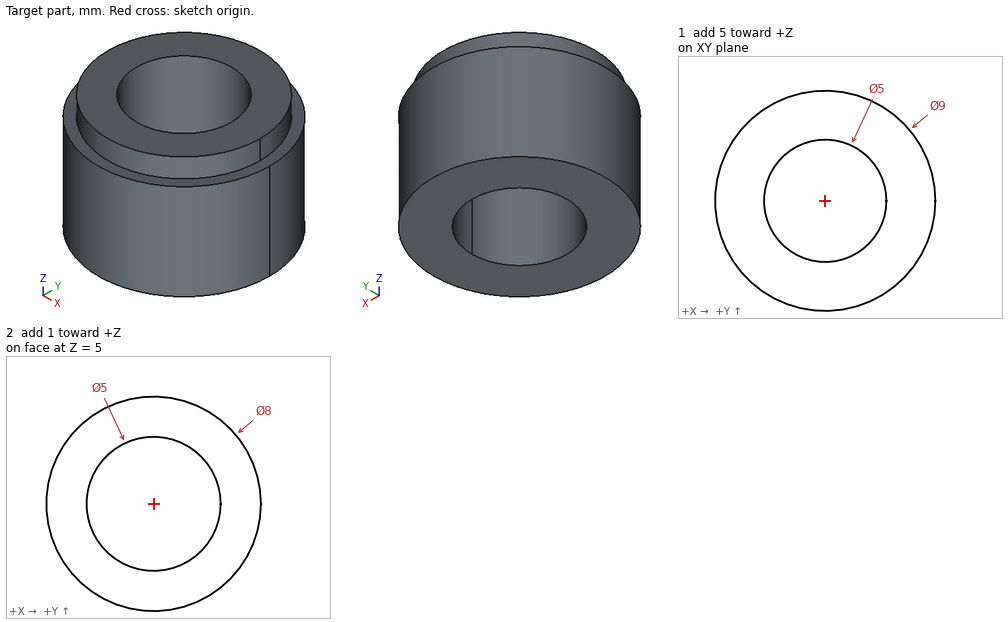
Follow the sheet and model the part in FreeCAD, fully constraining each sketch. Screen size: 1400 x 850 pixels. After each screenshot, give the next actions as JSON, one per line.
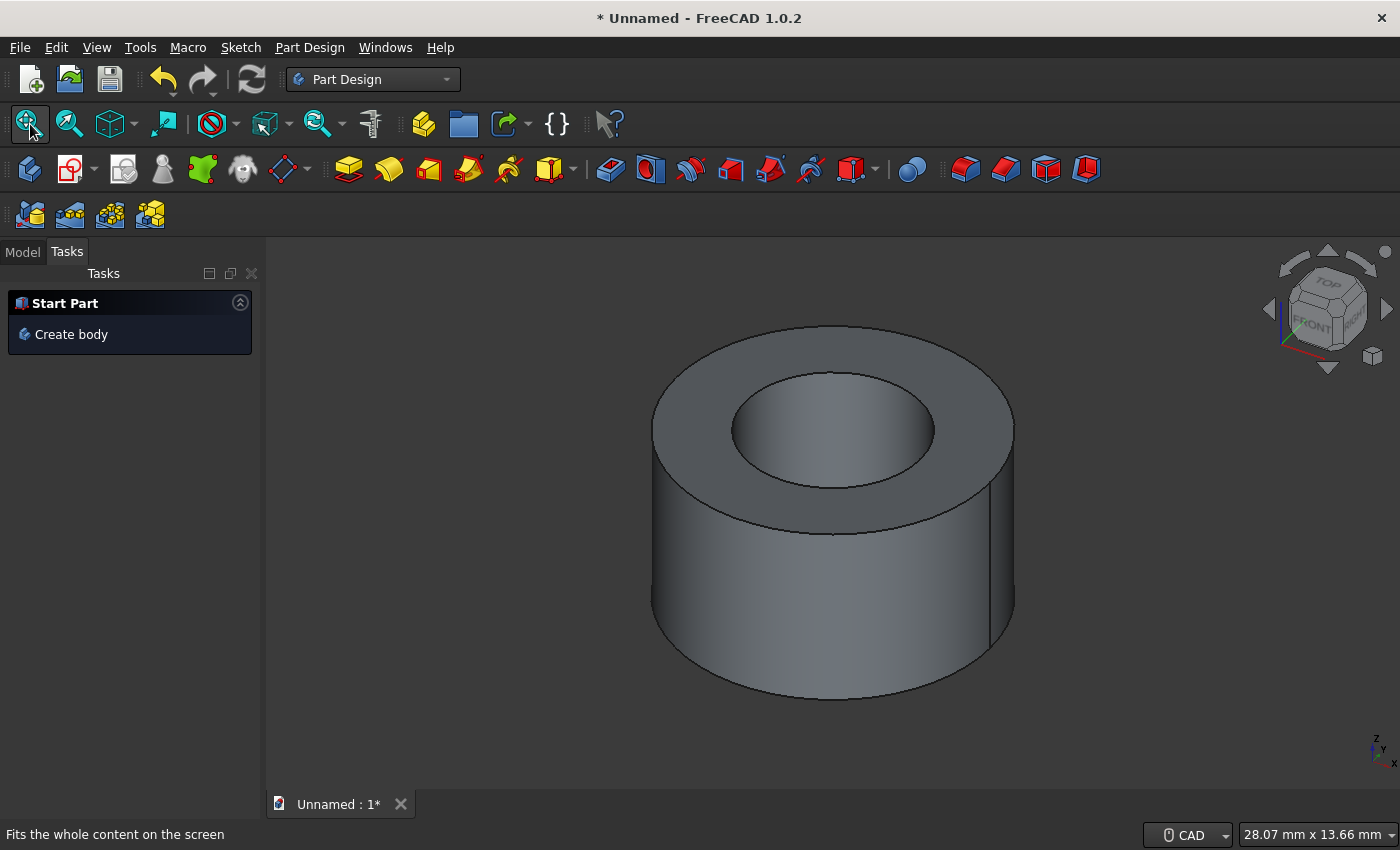
{"action": "left_click", "coordinate": [691, 451]}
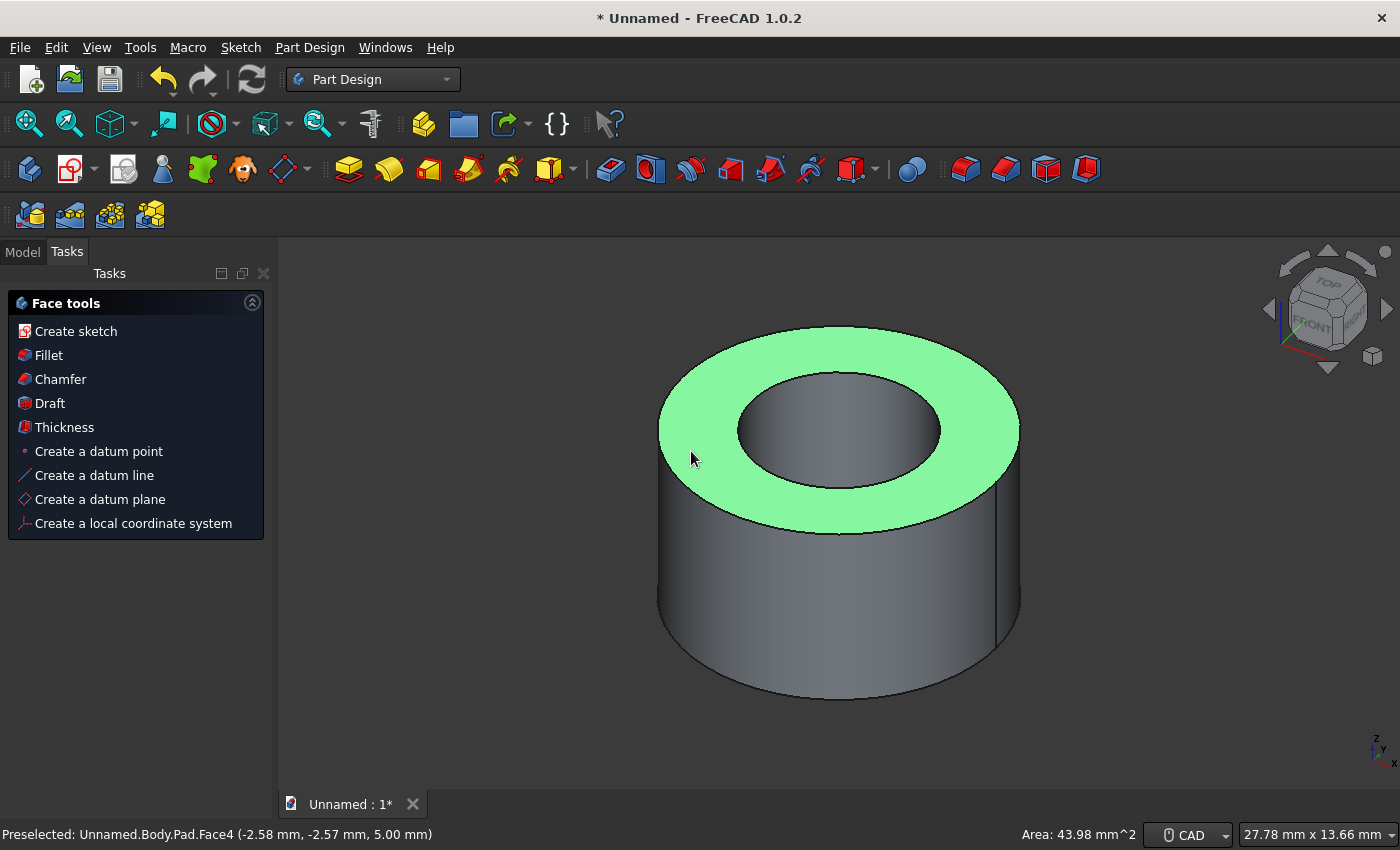
{"action": "left_click", "coordinate": [70, 170]}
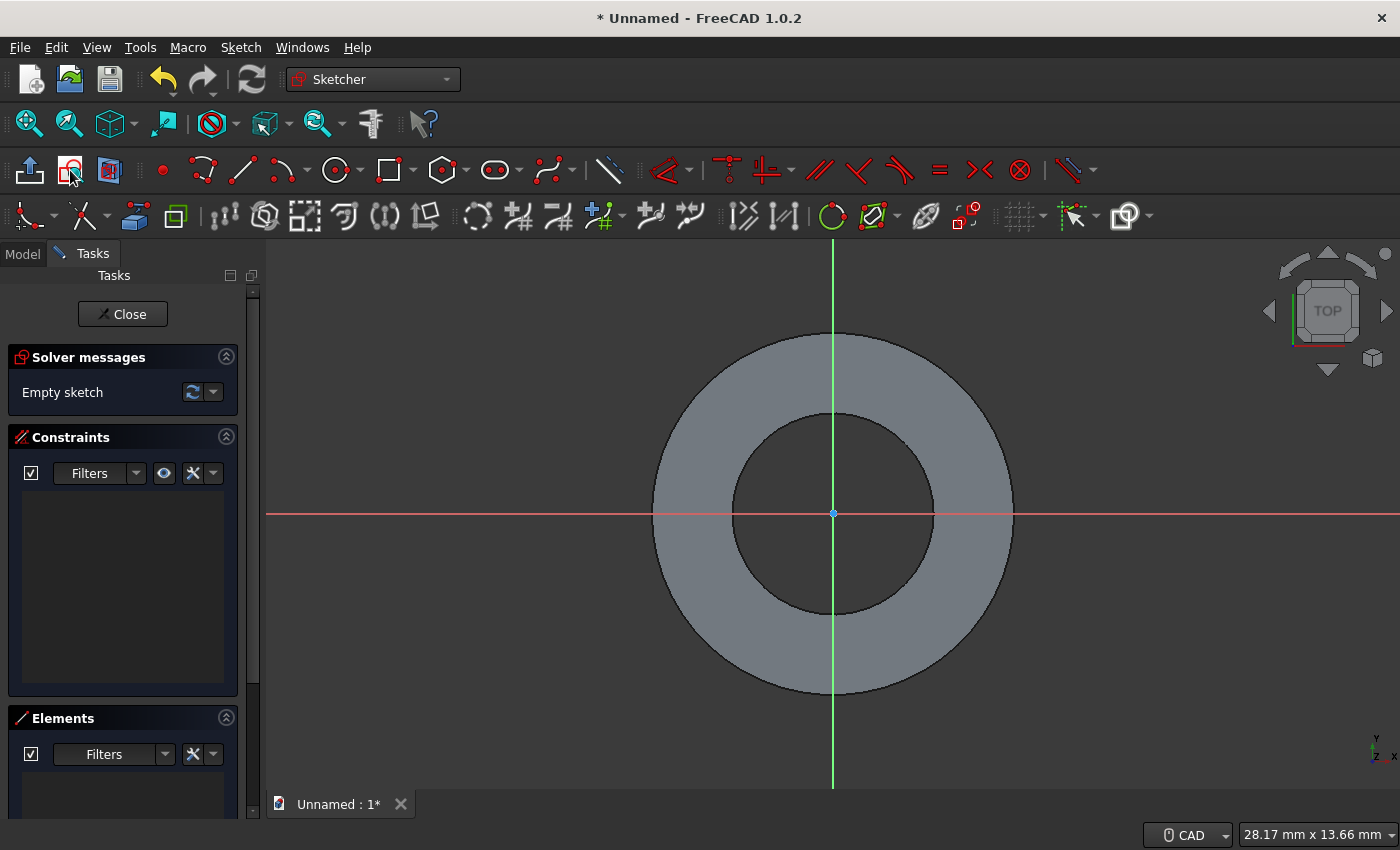
{"action": "left_click", "coordinate": [336, 170]}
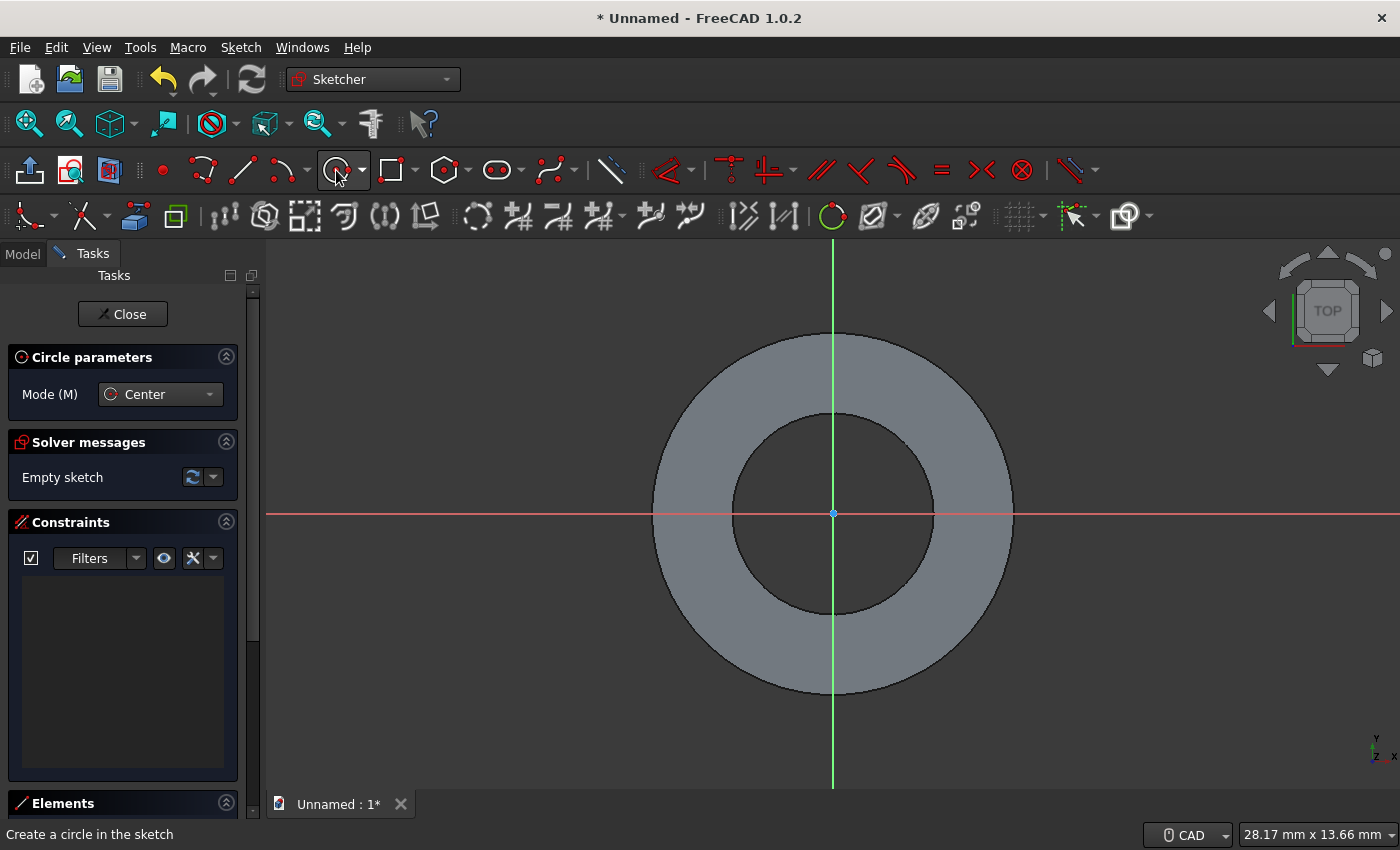
{"action": "left_click", "coordinate": [833, 514]}
{"action": "left_click", "coordinate": [947, 400]}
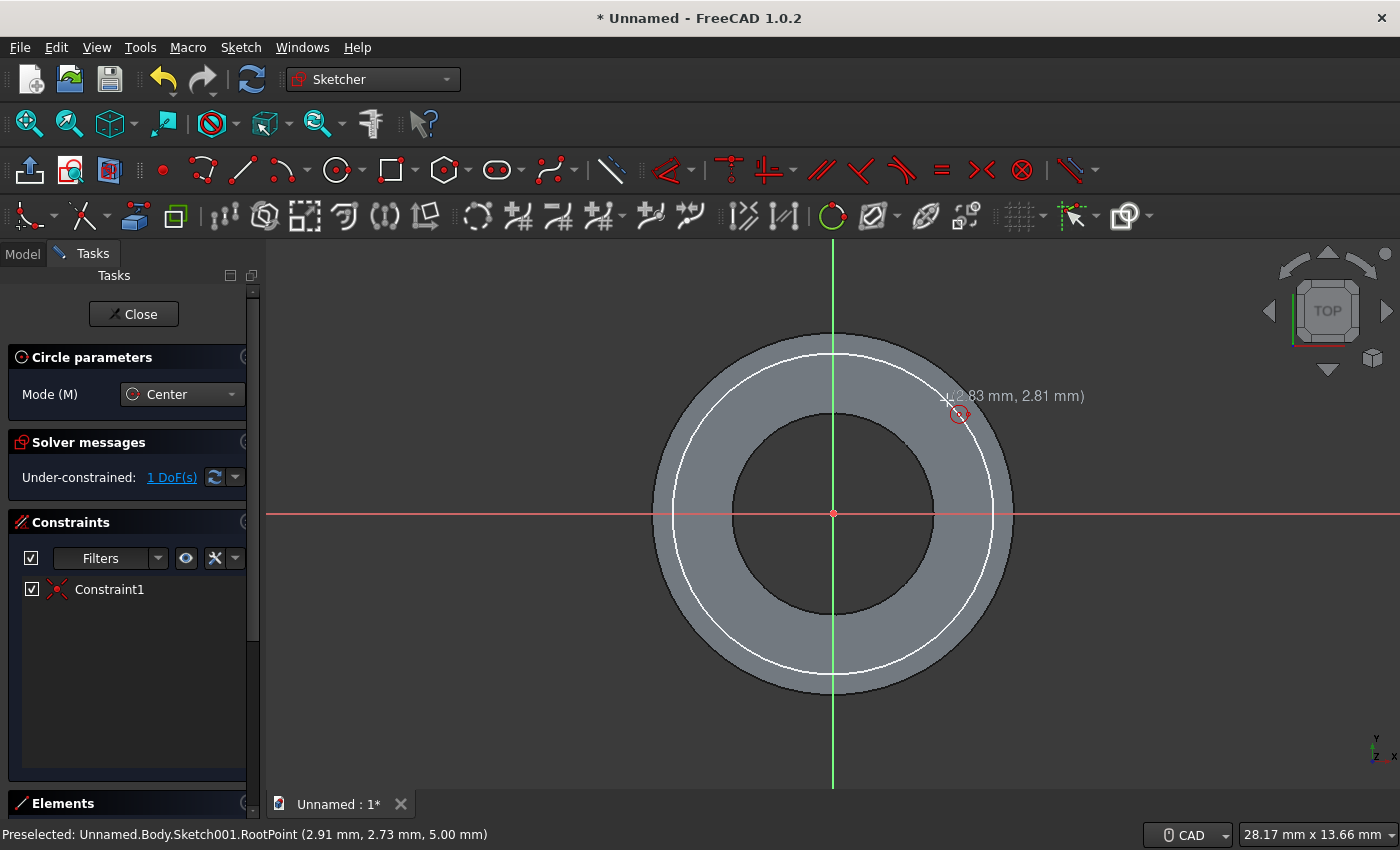
{"action": "left_click", "coordinate": [833, 514]}
{"action": "left_click", "coordinate": [904, 443]}
{"action": "key", "text": "Escape"}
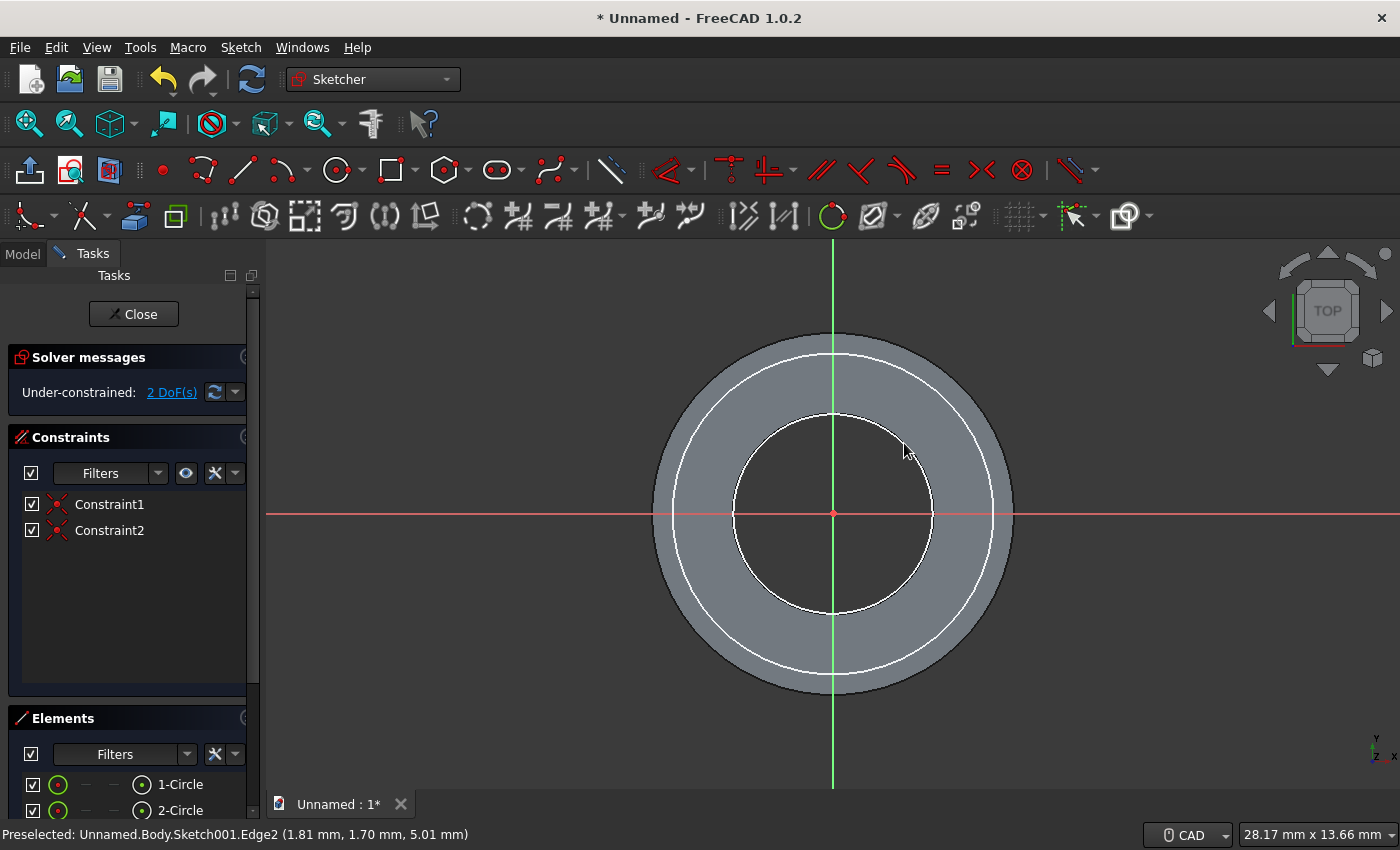
{"action": "left_click", "coordinate": [666, 170]}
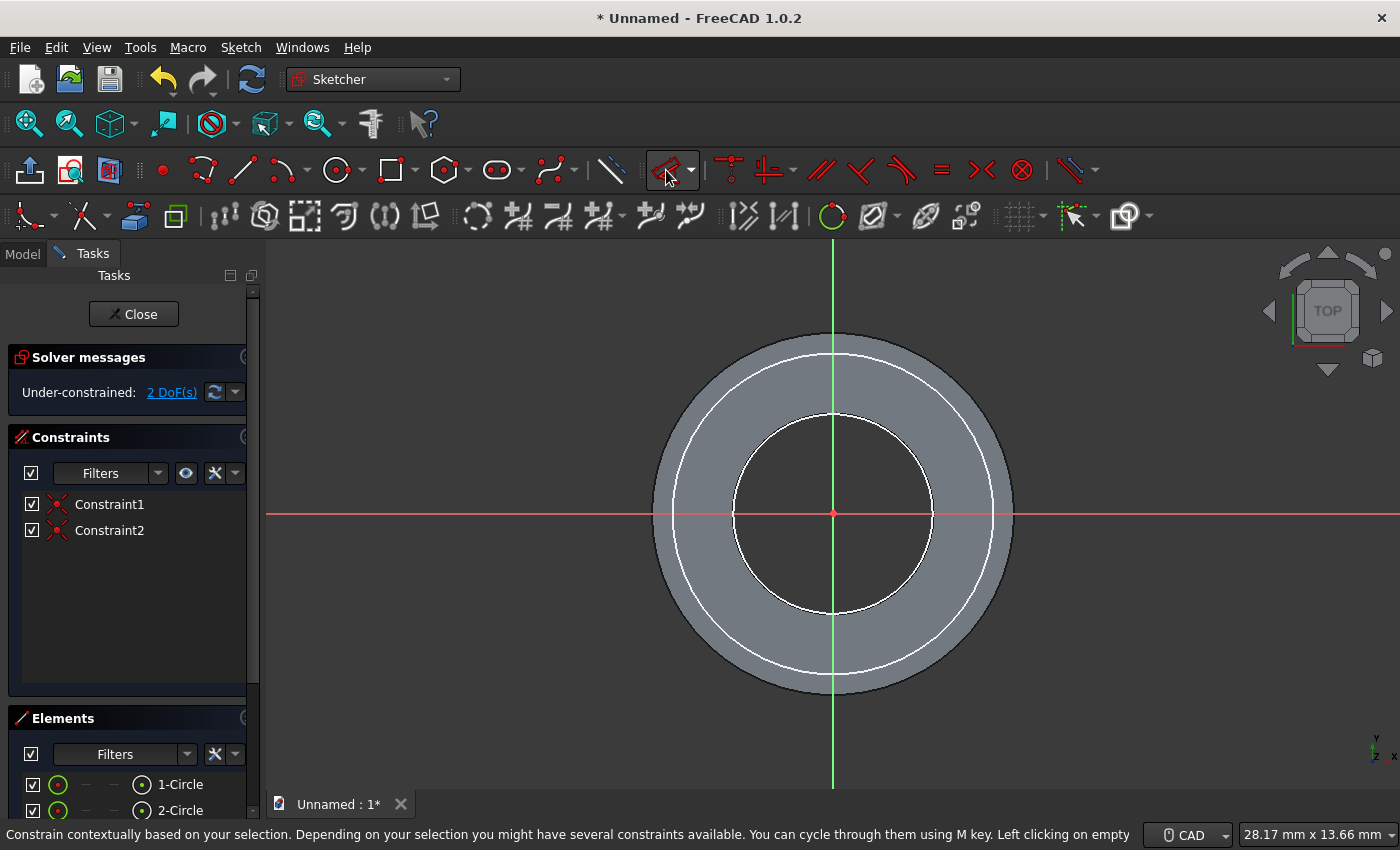
{"action": "left_click", "coordinate": [946, 400]}
{"action": "left_click", "coordinate": [969, 377]}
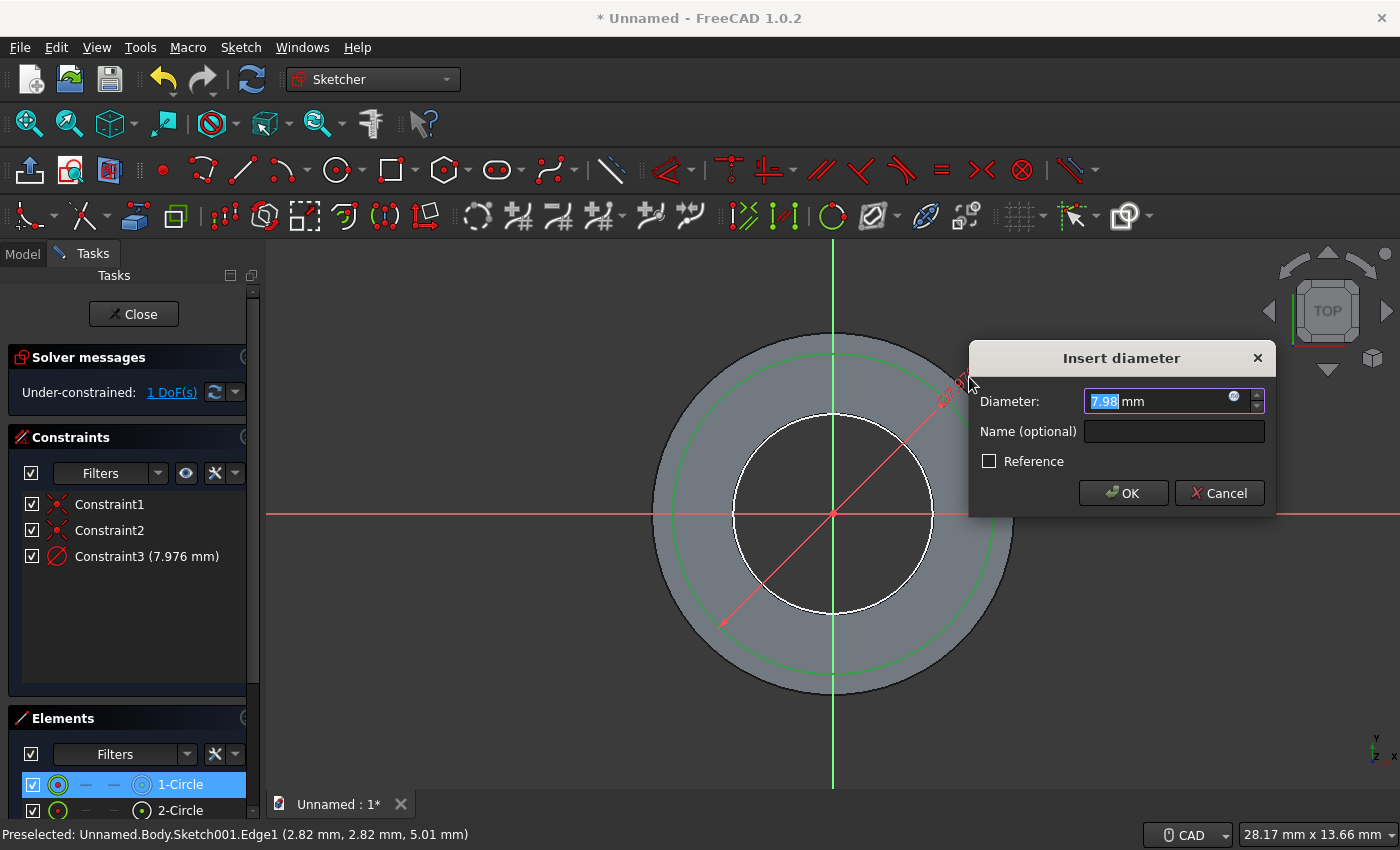
{"action": "type", "text": "8"}
{"action": "key", "text": "Return"}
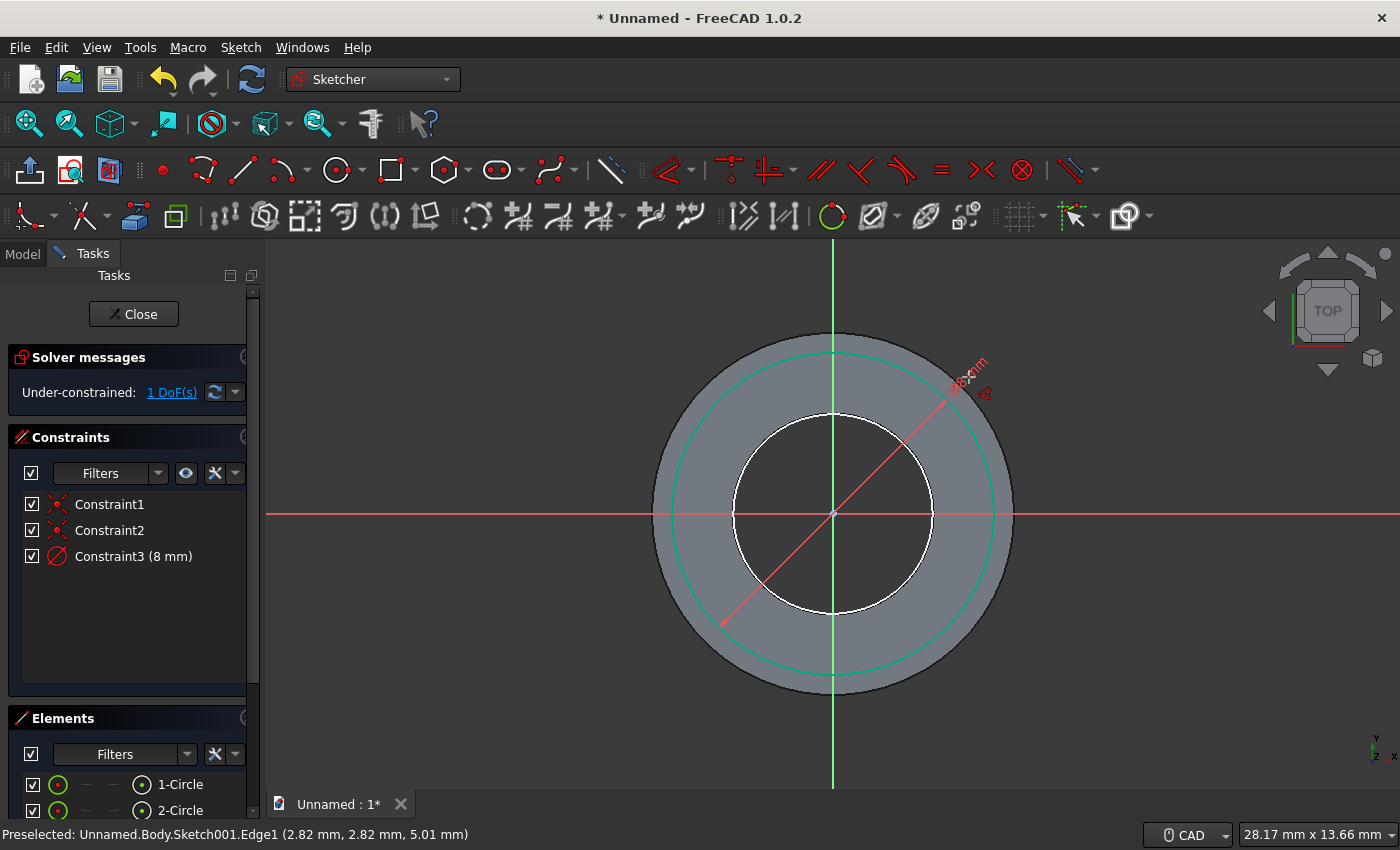
{"action": "left_click", "coordinate": [903, 443]}
{"action": "left_click", "coordinate": [925, 420]}